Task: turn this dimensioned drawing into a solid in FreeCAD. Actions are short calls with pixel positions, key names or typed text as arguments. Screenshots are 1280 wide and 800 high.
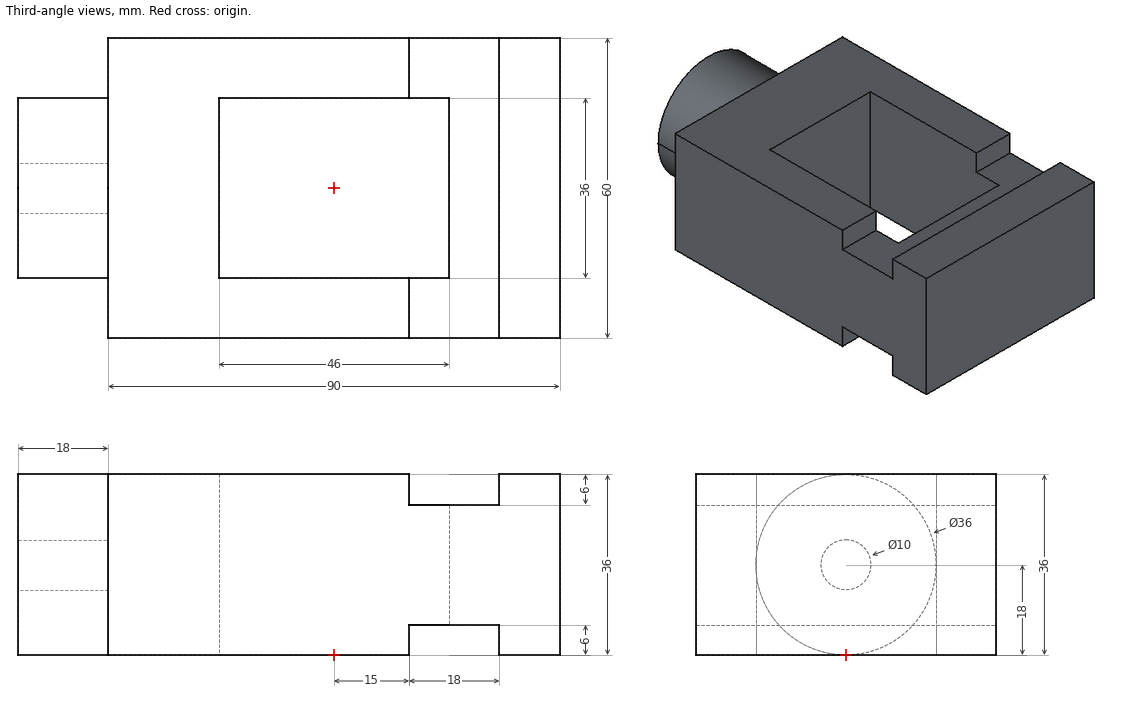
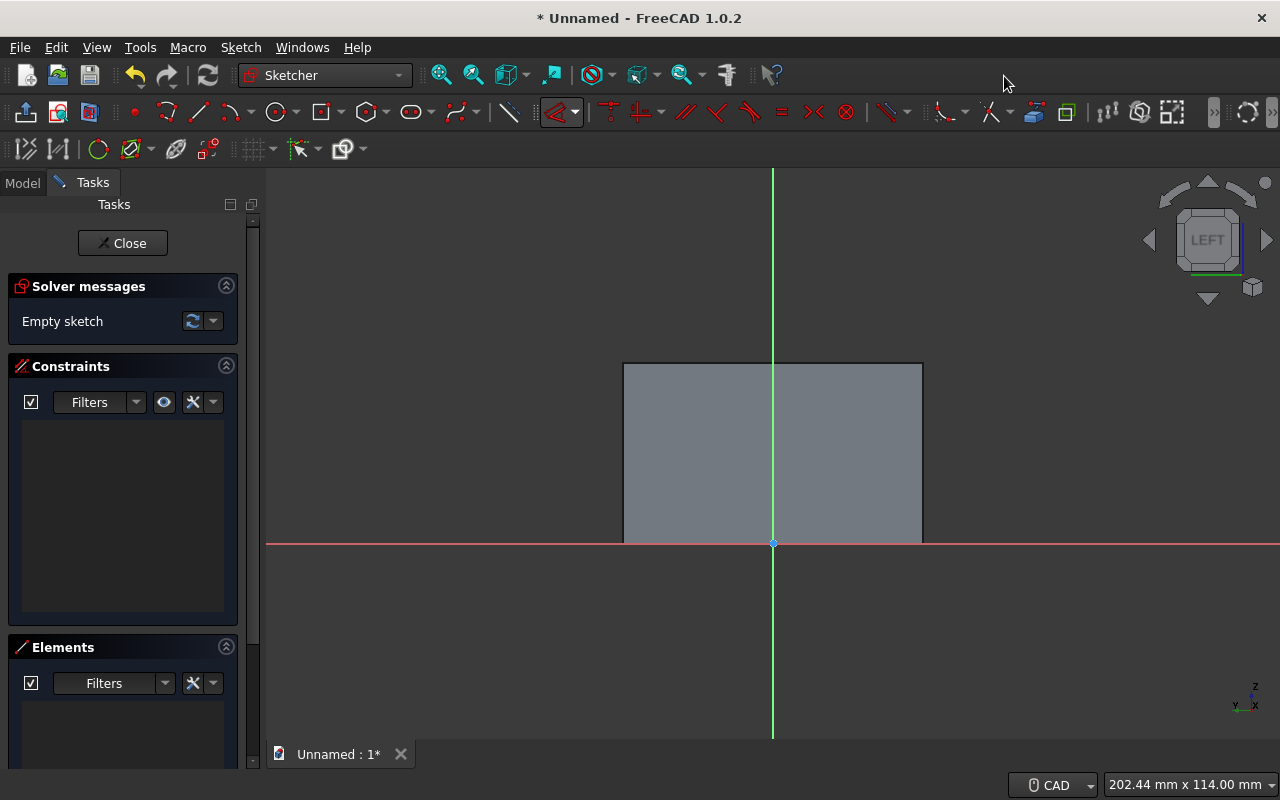
scroll(829, 454, up, 4)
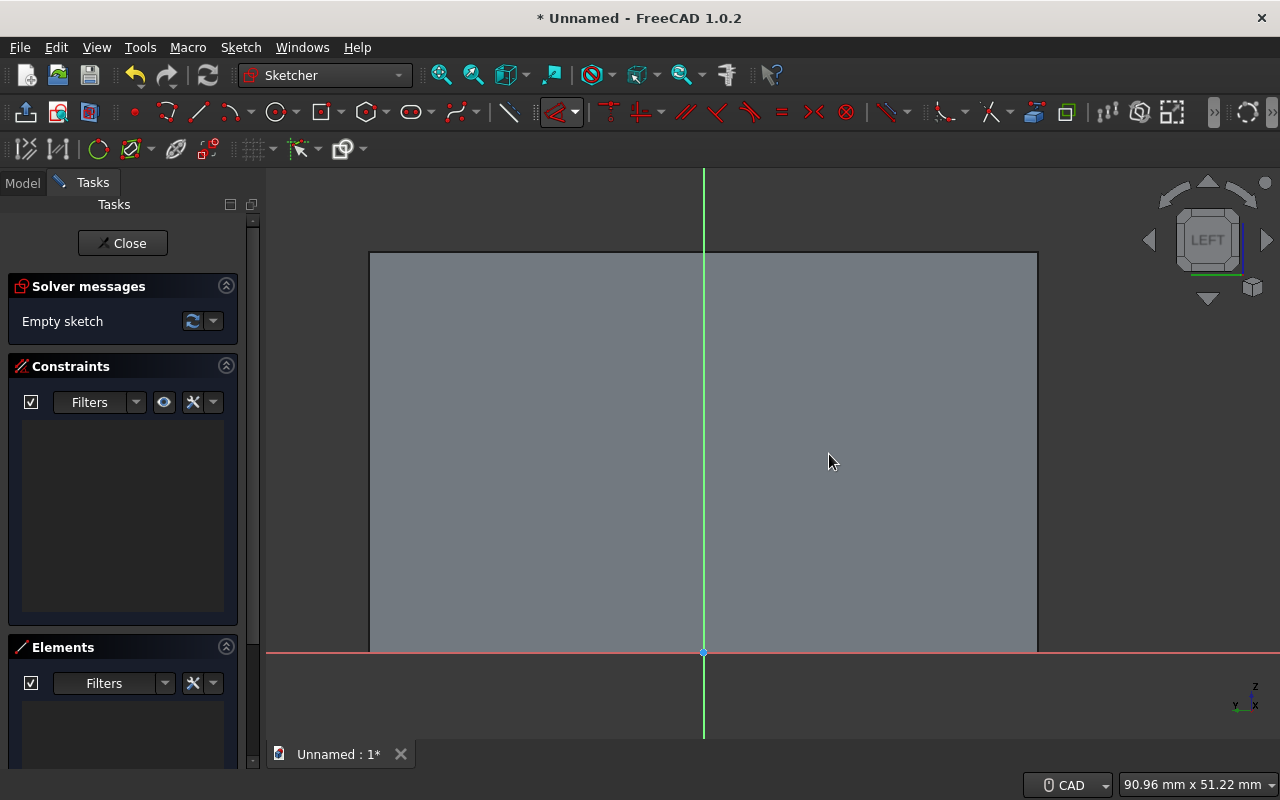
click(276, 112)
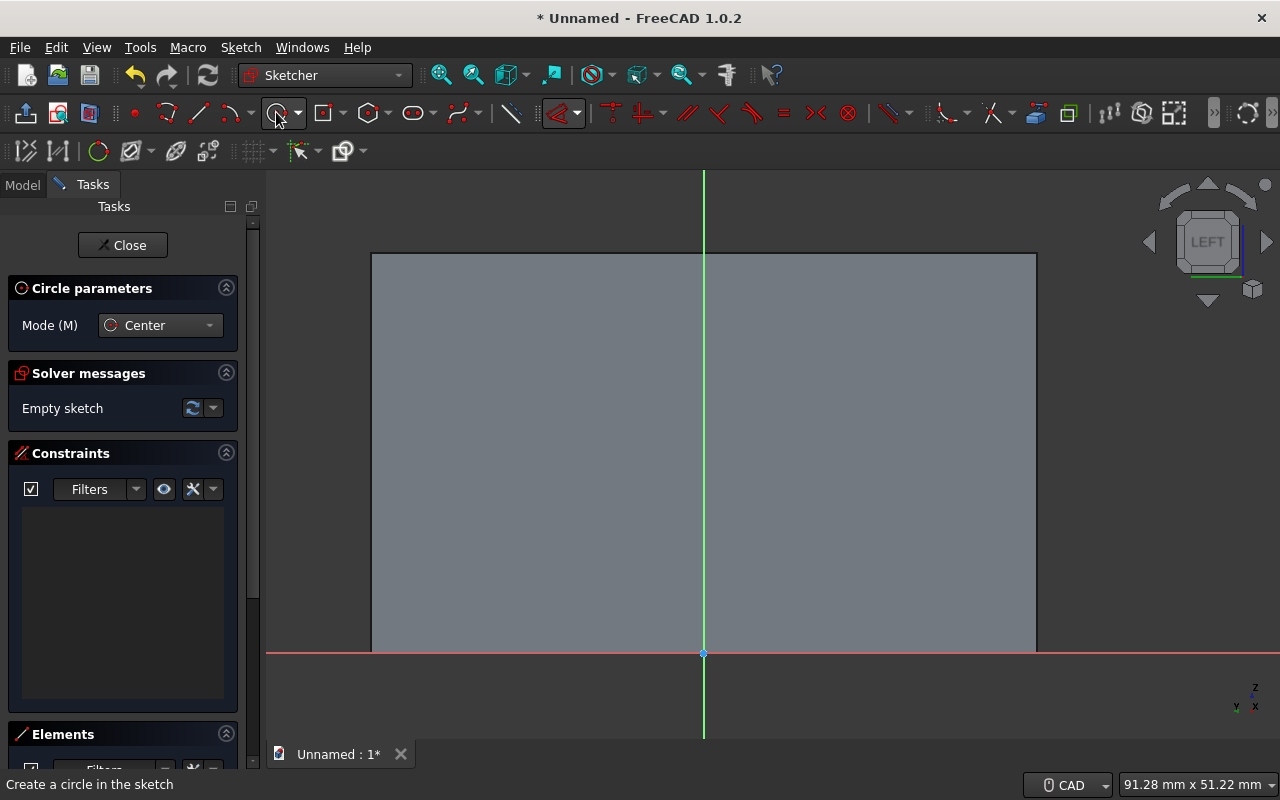
click(704, 453)
click(845, 312)
key(Escape)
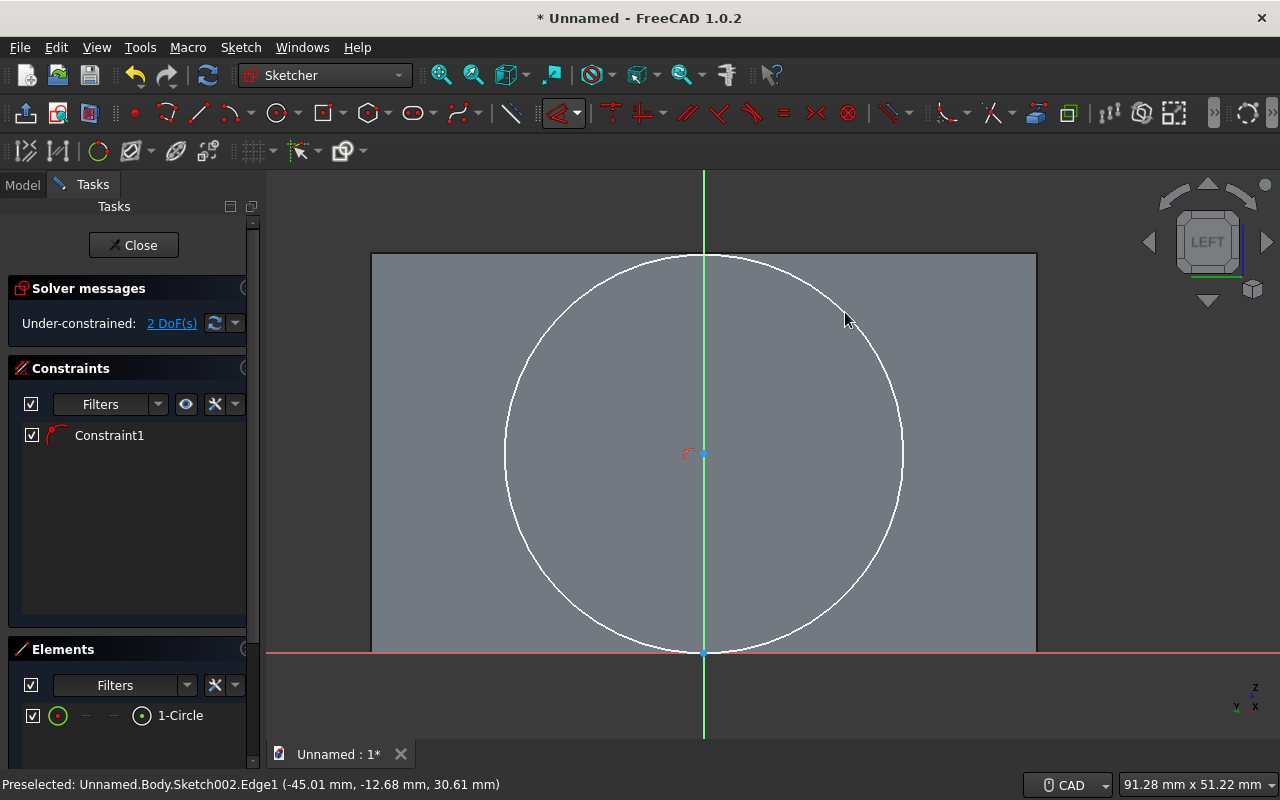
click(845, 313)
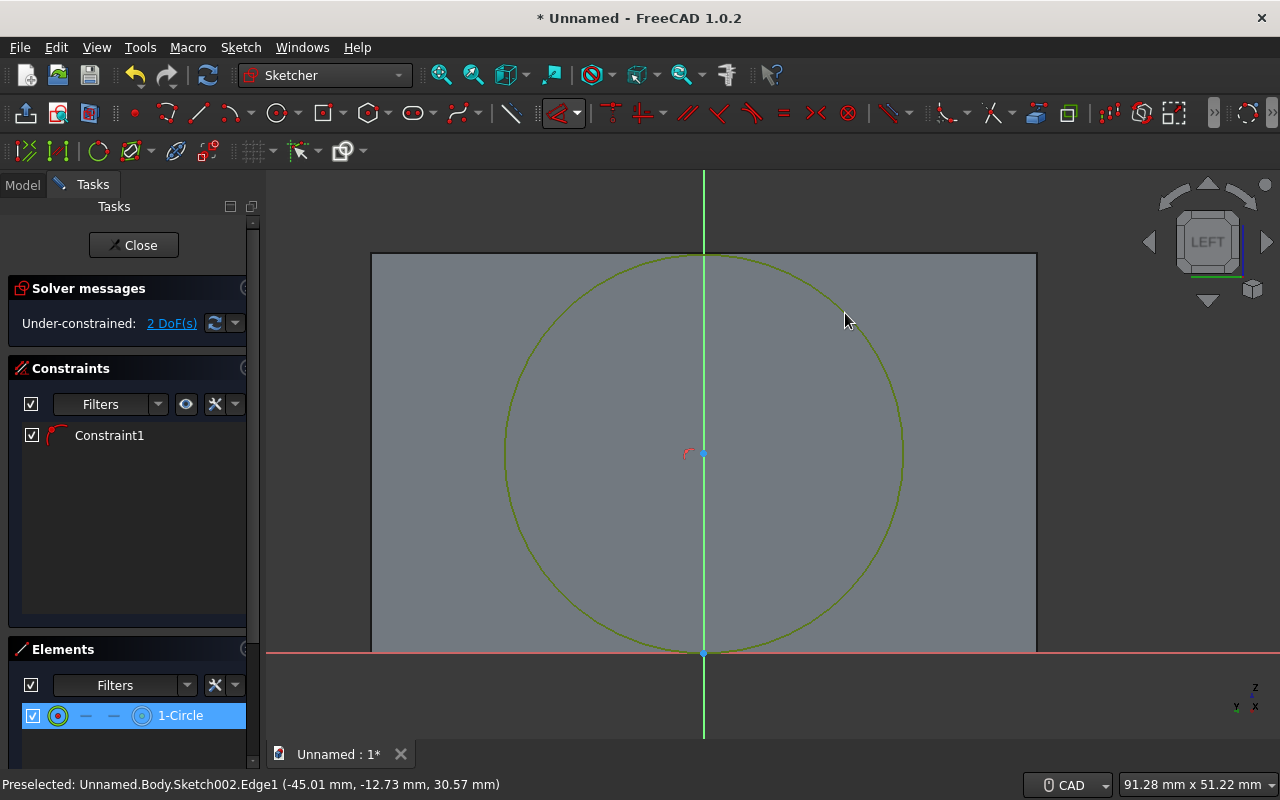
click(580, 114)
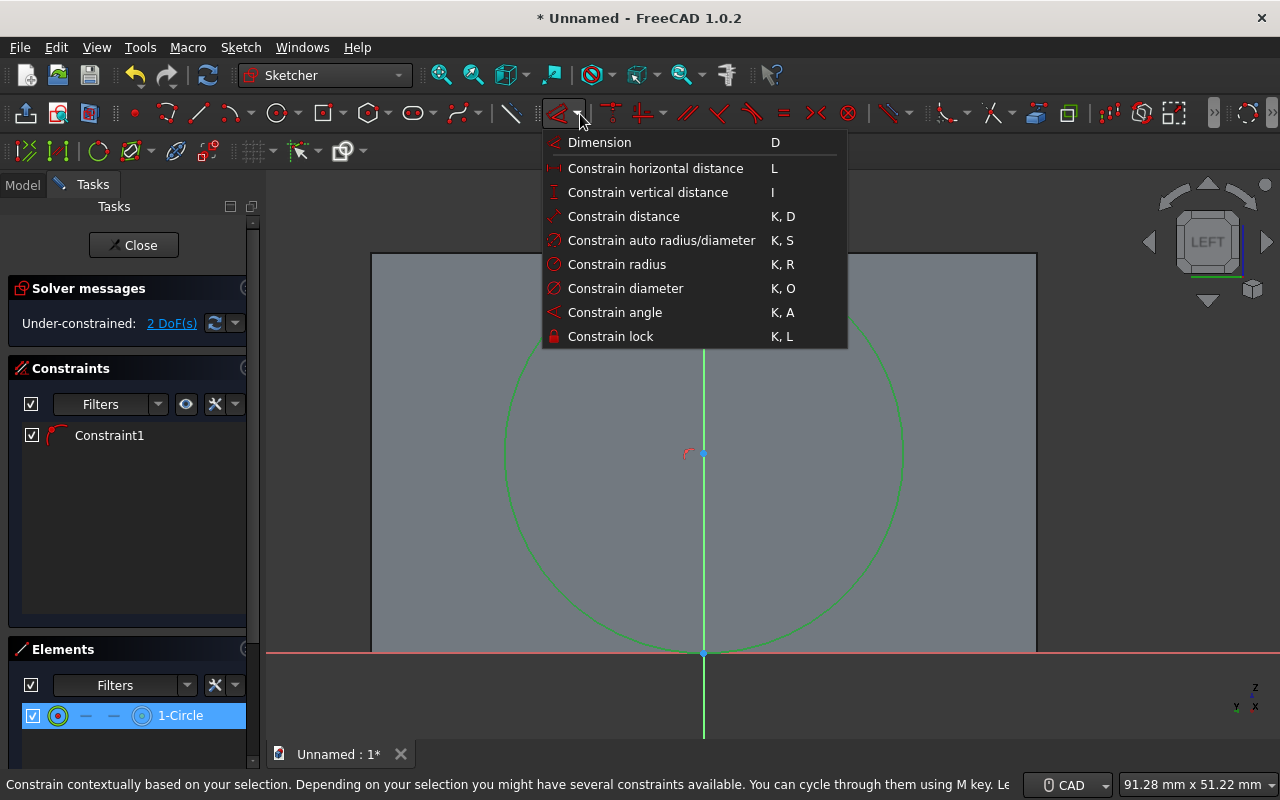
click(695, 288)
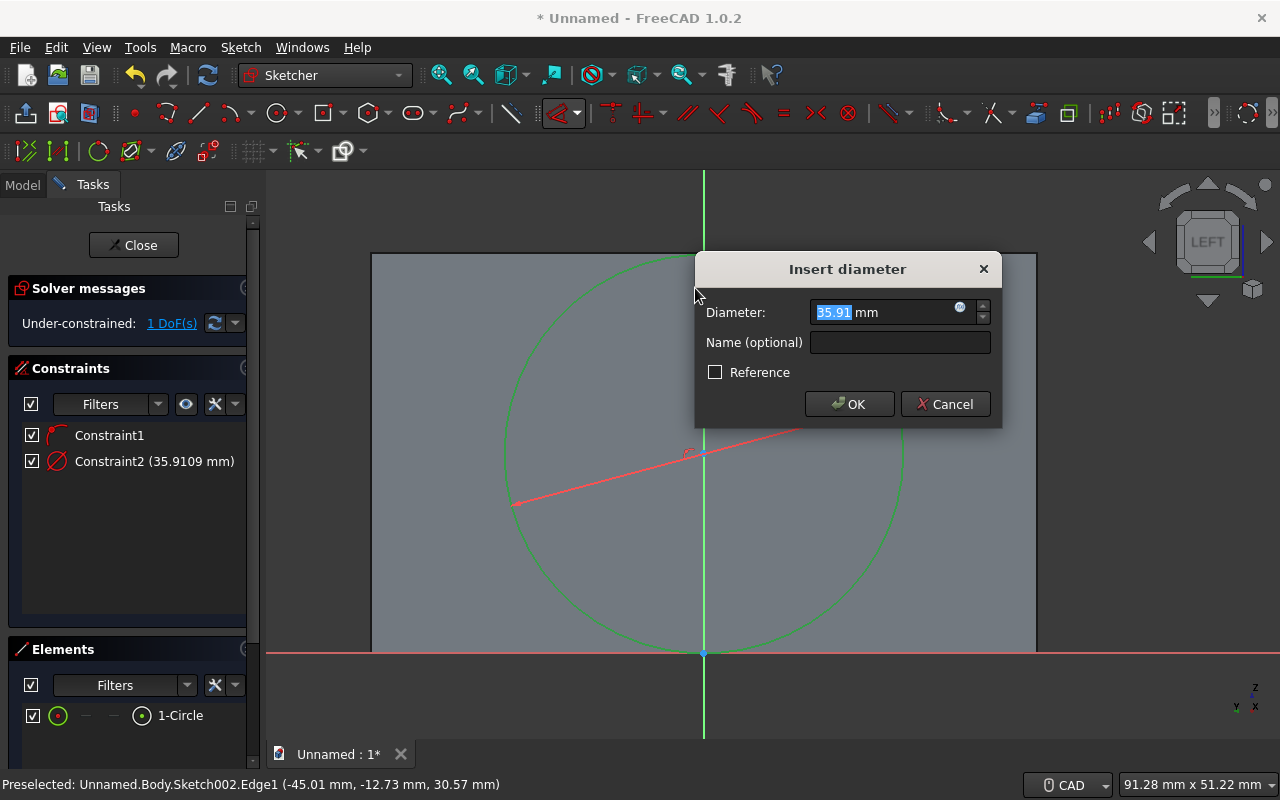
text(36)
key(Return)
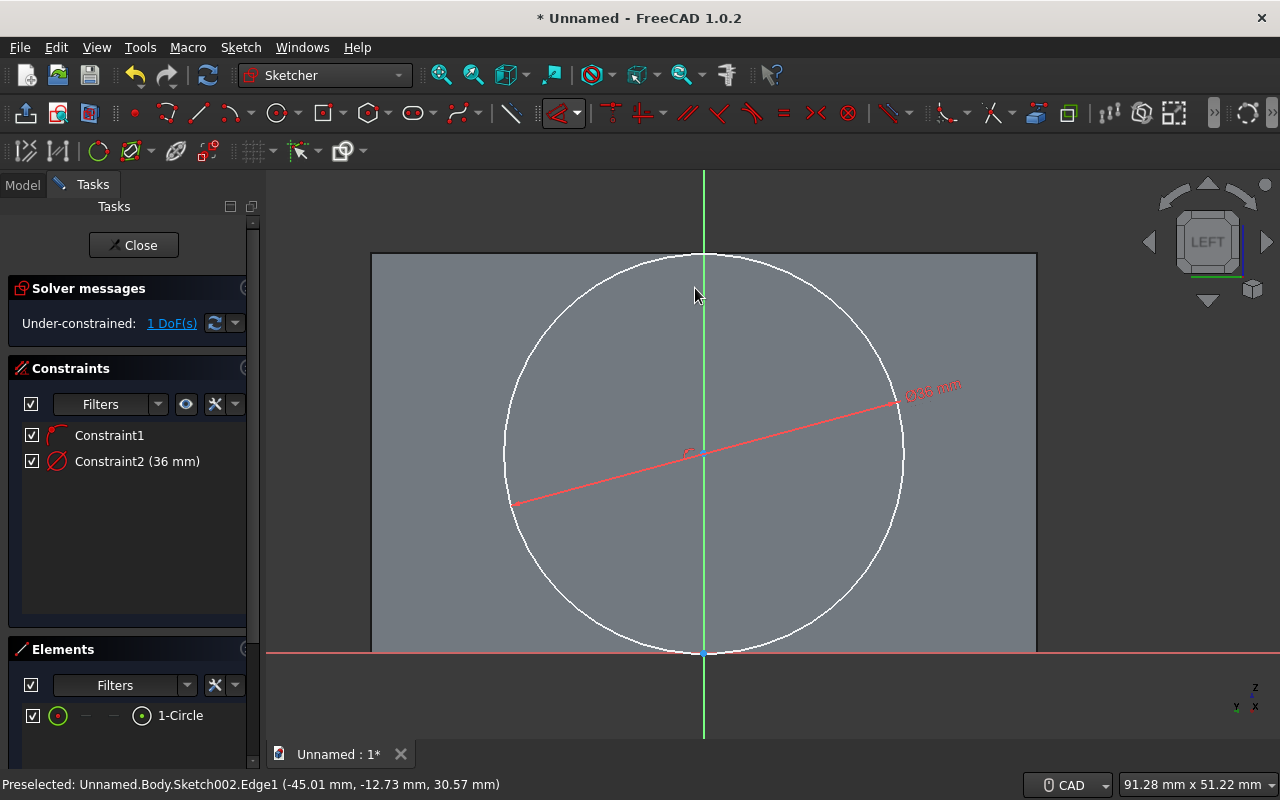
click(704, 454)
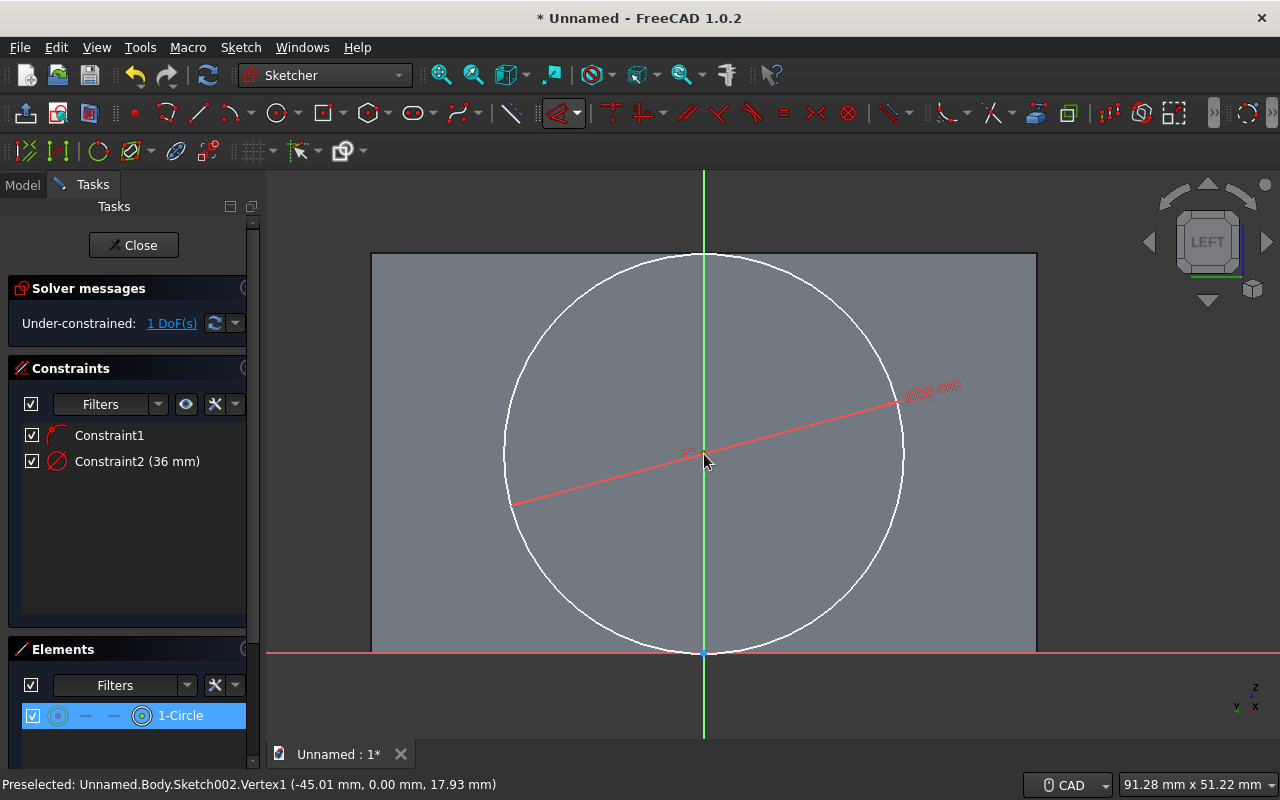
click(580, 114)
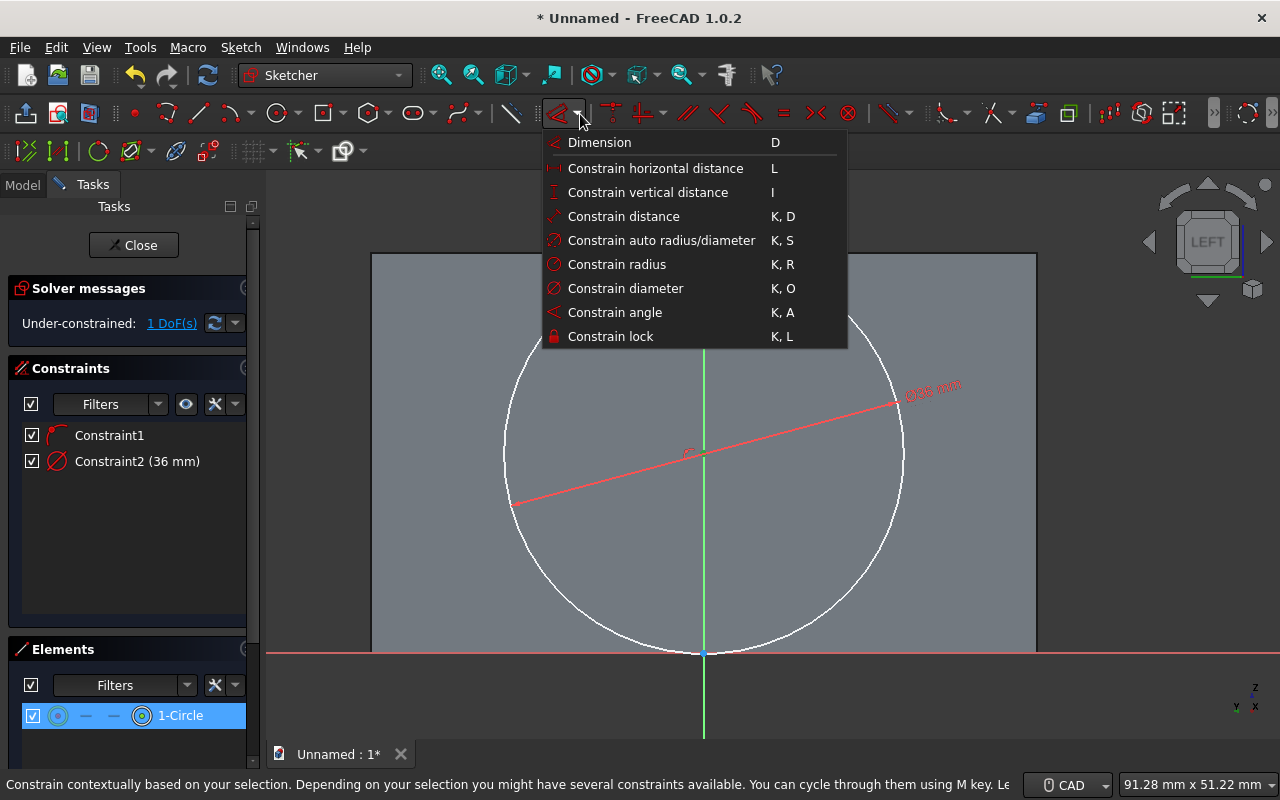
click(695, 192)